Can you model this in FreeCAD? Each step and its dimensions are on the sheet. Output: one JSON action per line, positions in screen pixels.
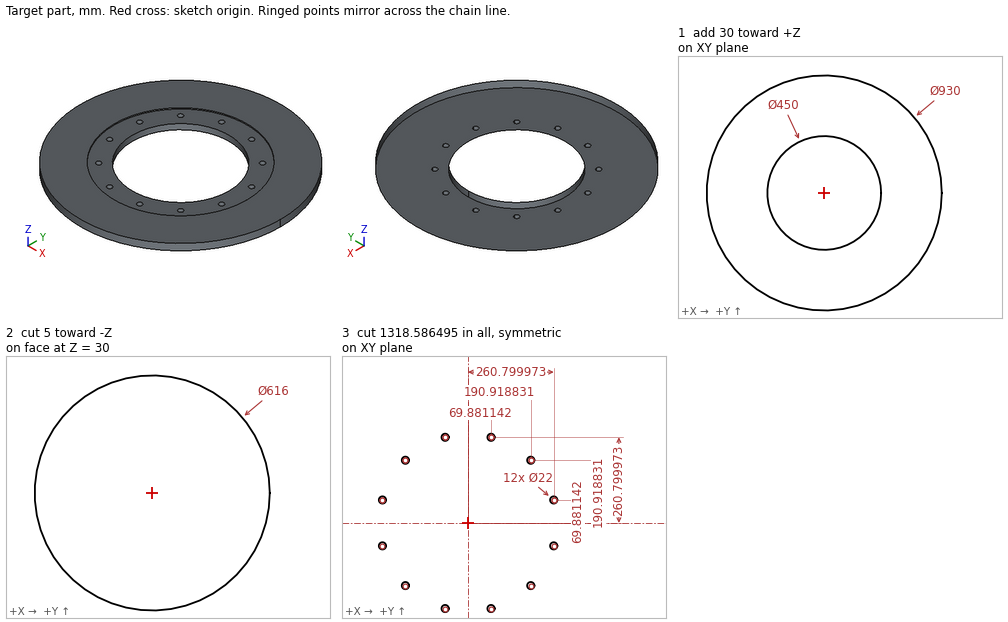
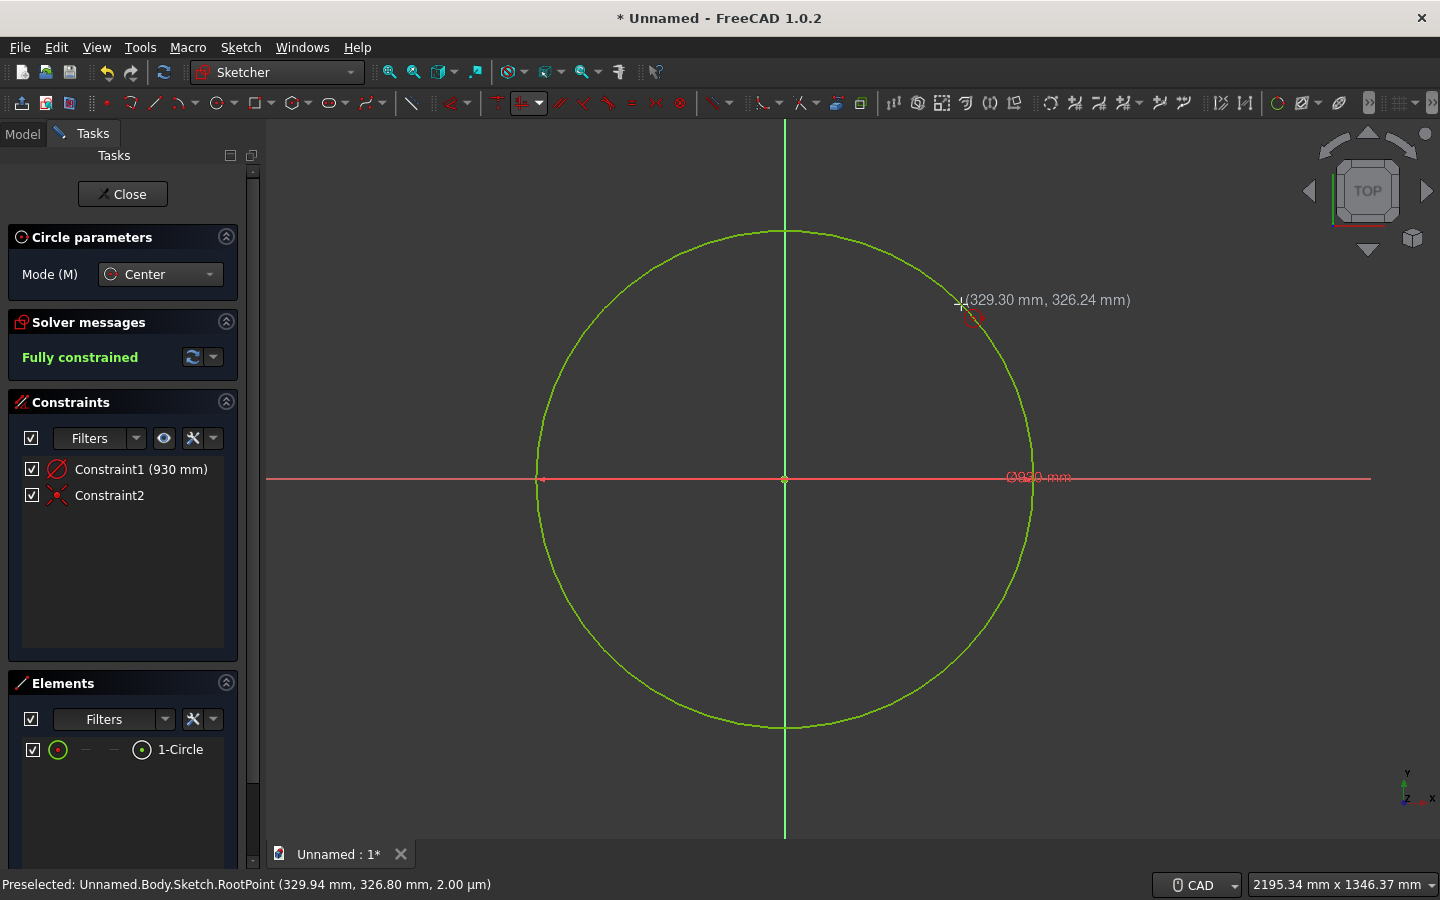
{"action": "left_click", "coordinate": [785, 479]}
{"action": "mouse_move", "coordinate": [870, 394]}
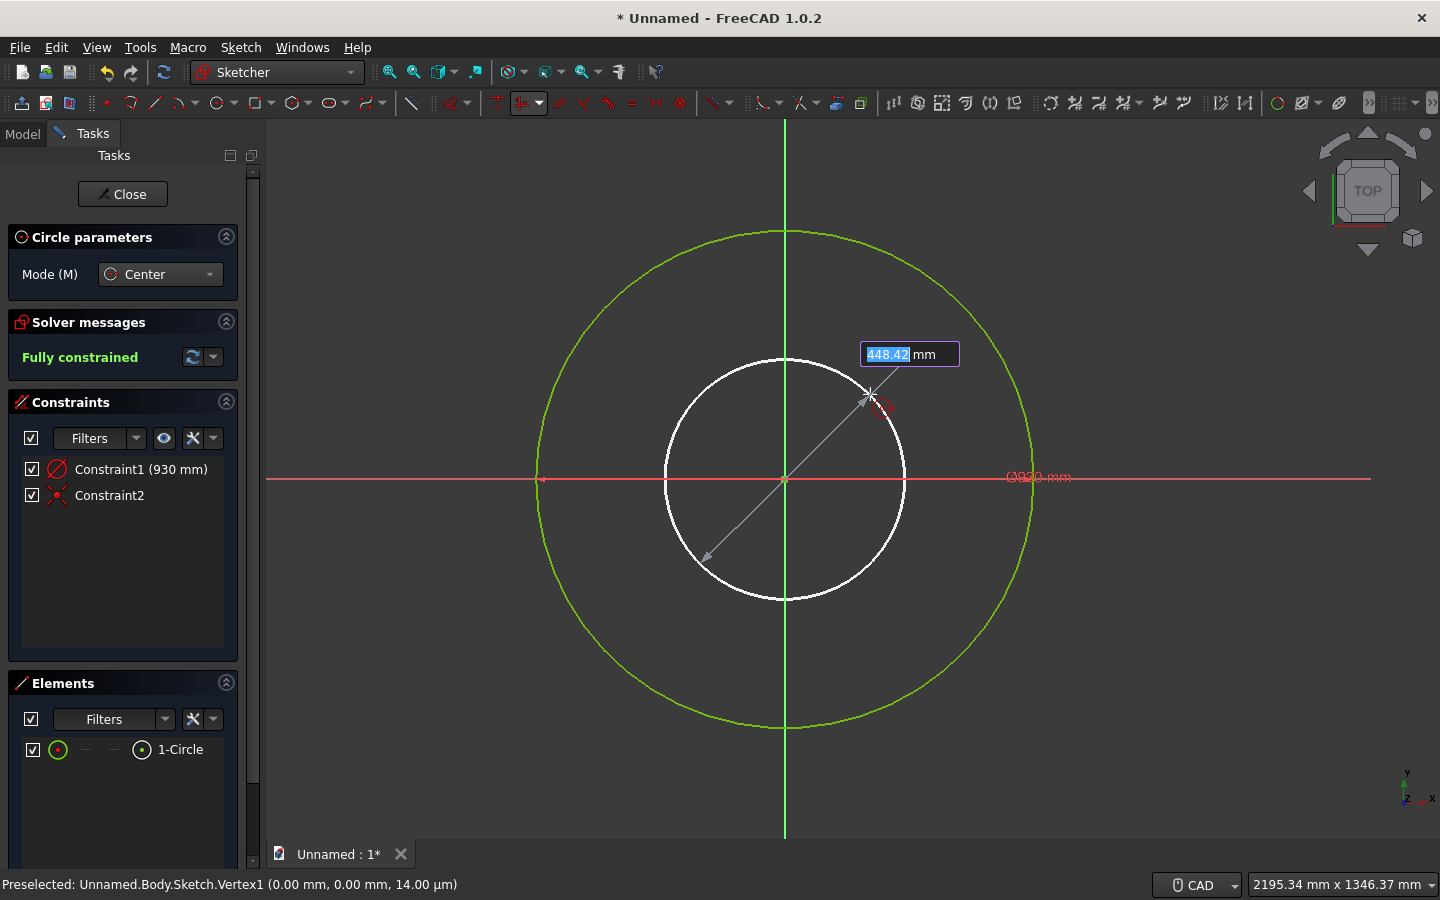
{"action": "type", "text": "450"}
{"action": "key", "text": "Return"}
{"action": "key", "text": "Escape"}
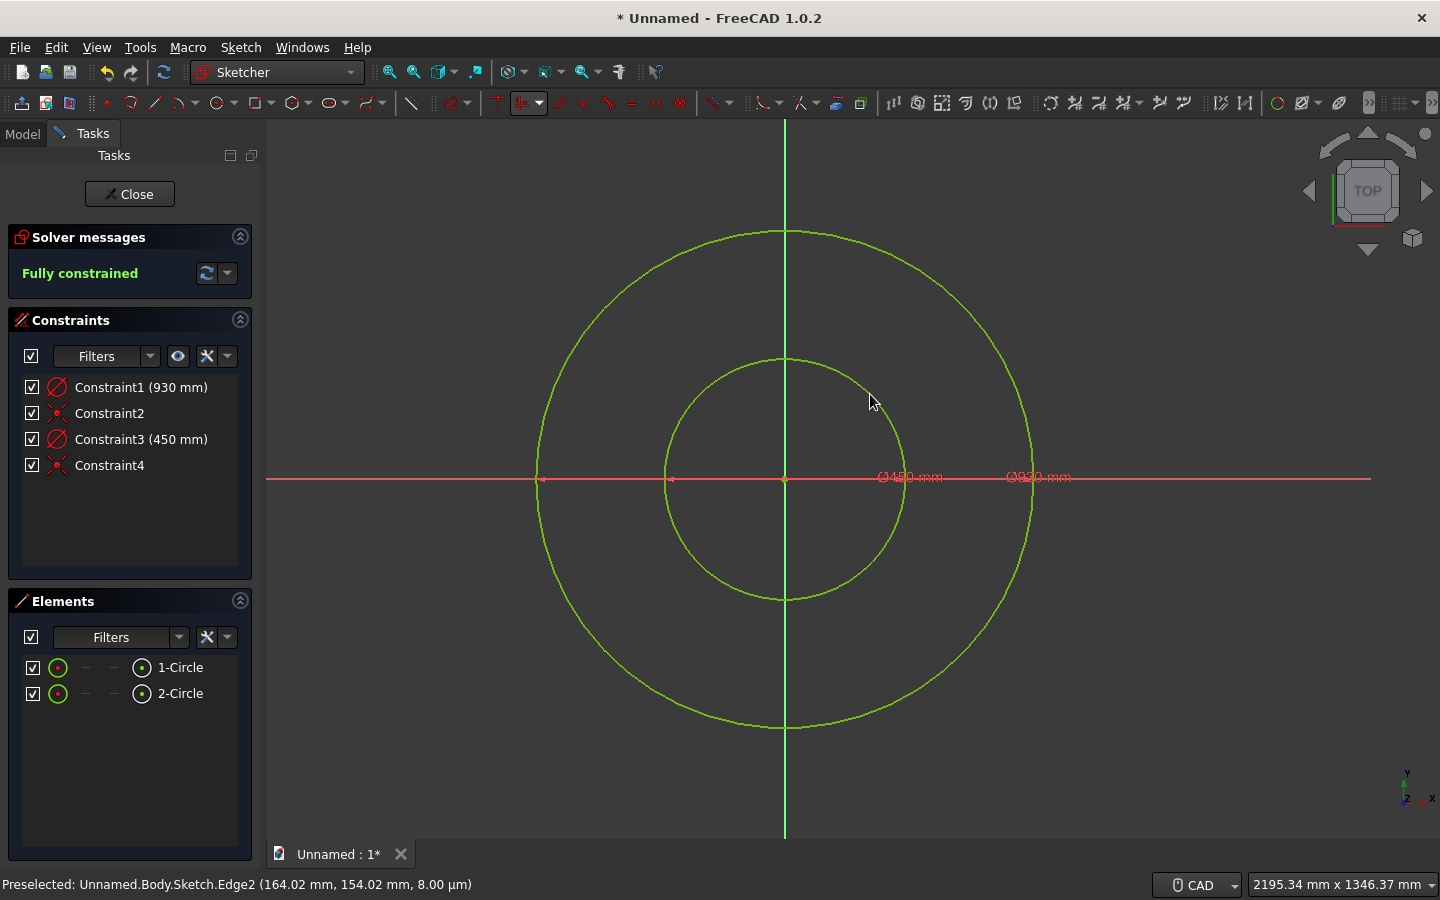
{"action": "left_click", "coordinate": [130, 194]}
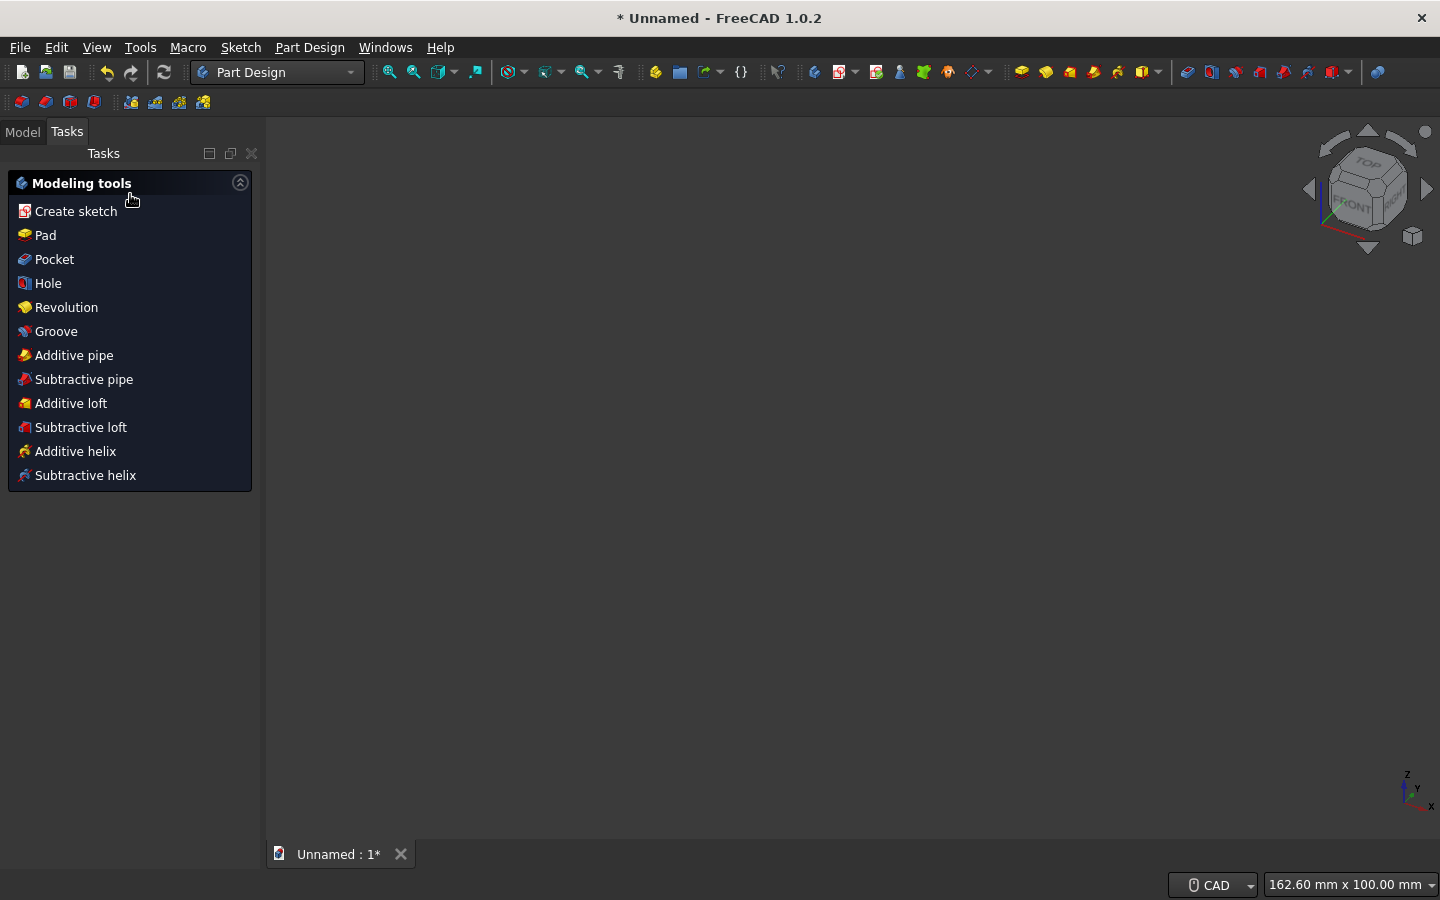
{"action": "left_click", "coordinate": [1022, 72]}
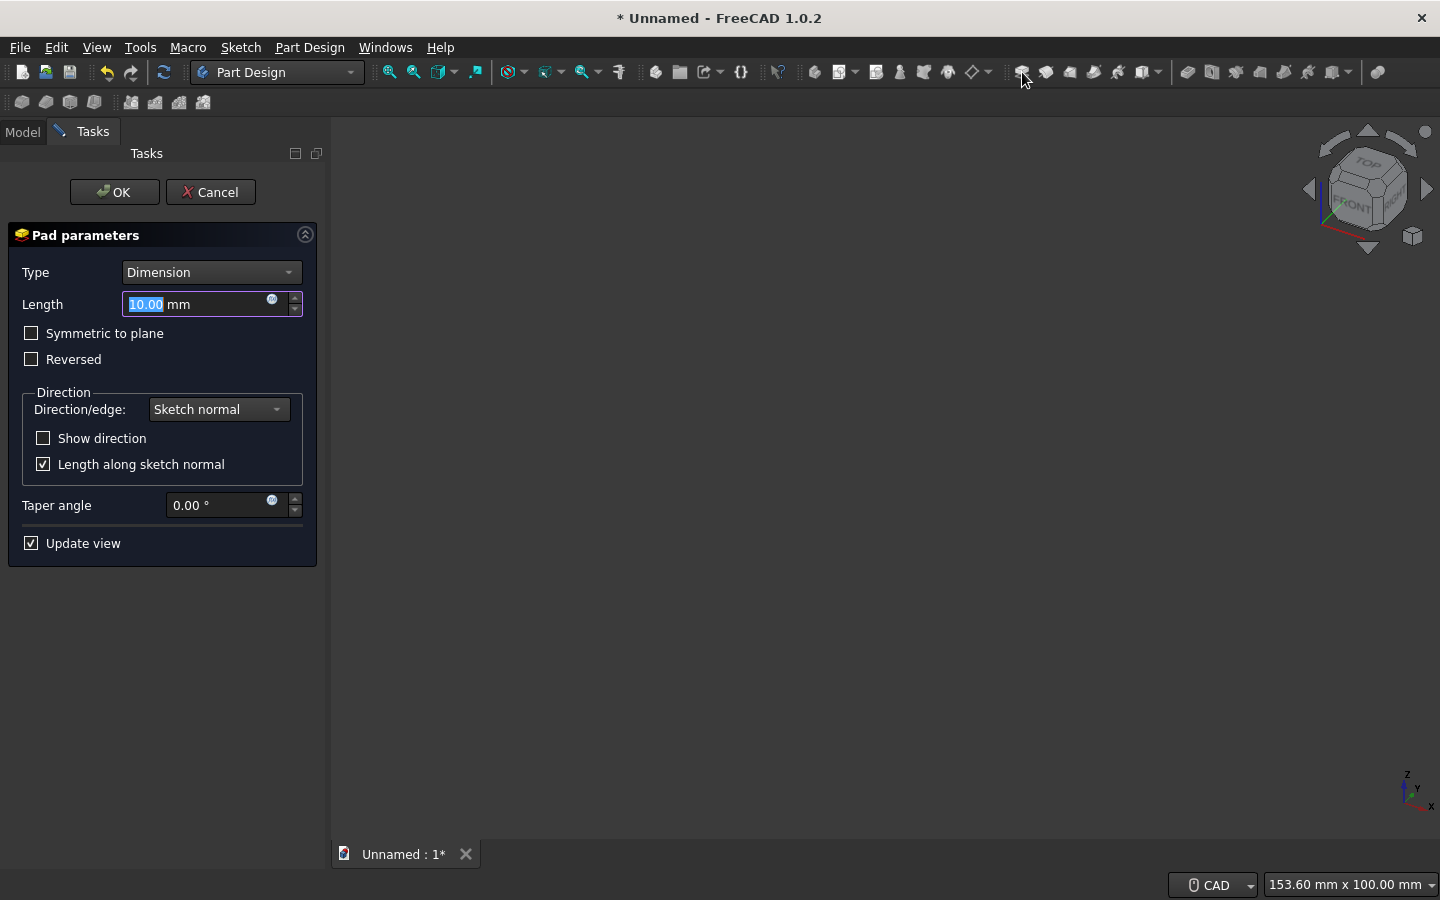
{"action": "type", "text": "30"}
{"action": "key", "text": "Tab"}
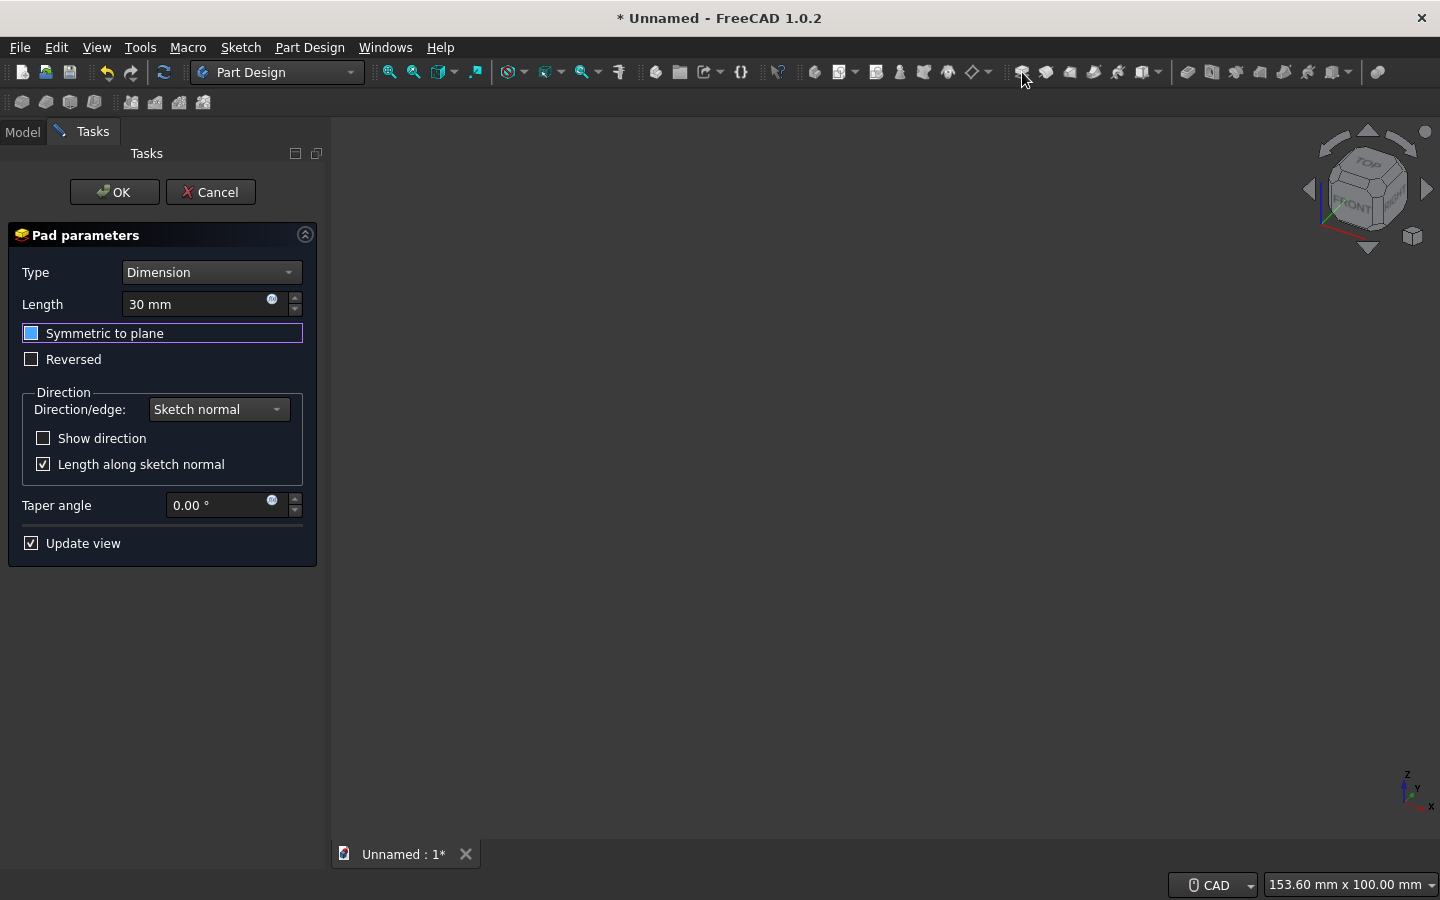
{"action": "left_click", "coordinate": [115, 192]}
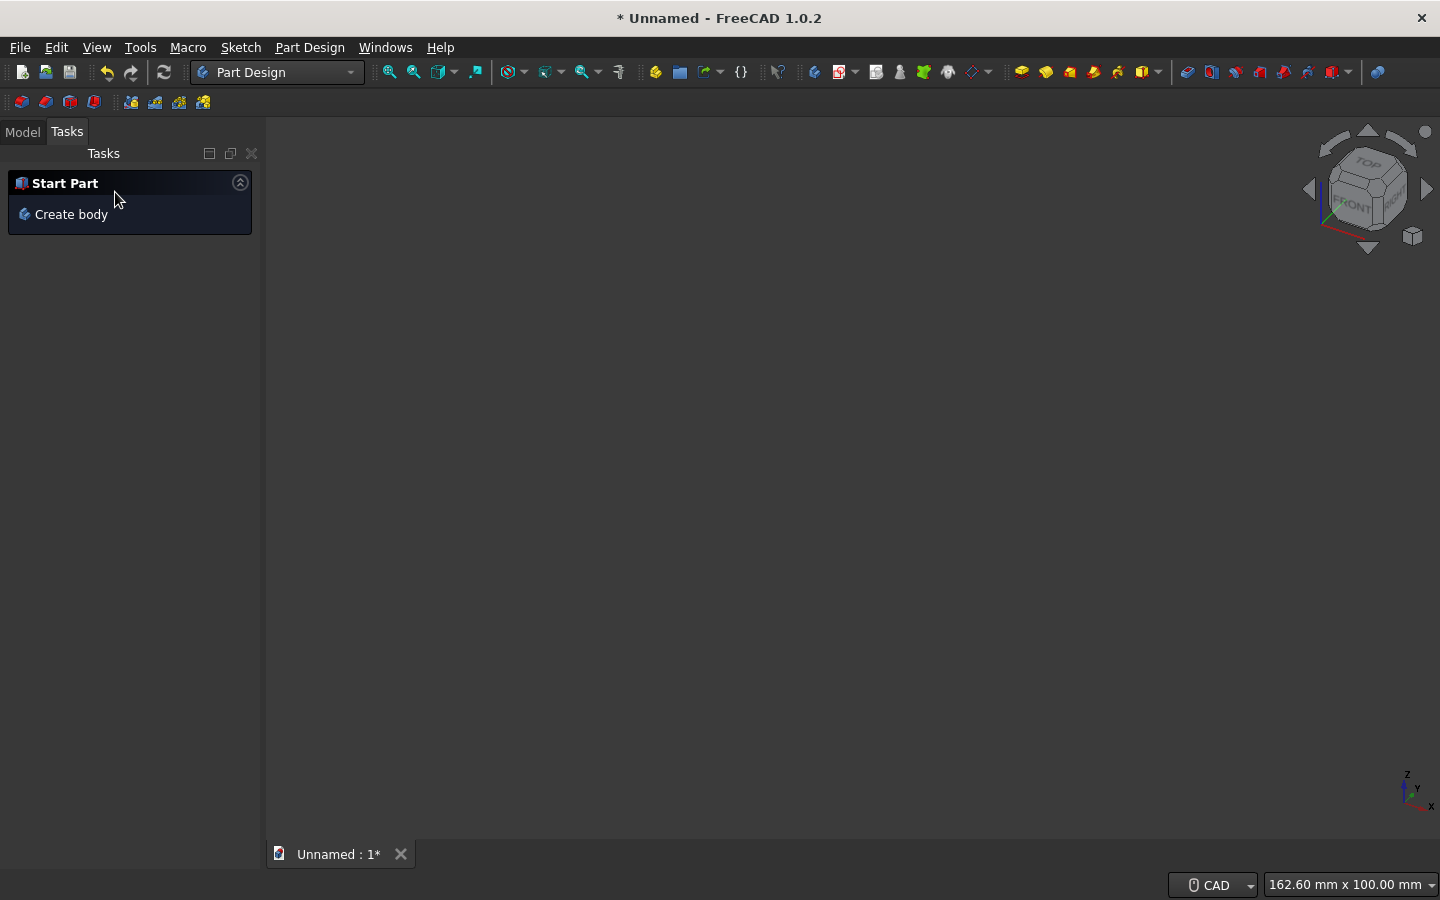
{"action": "left_click", "coordinate": [390, 72]}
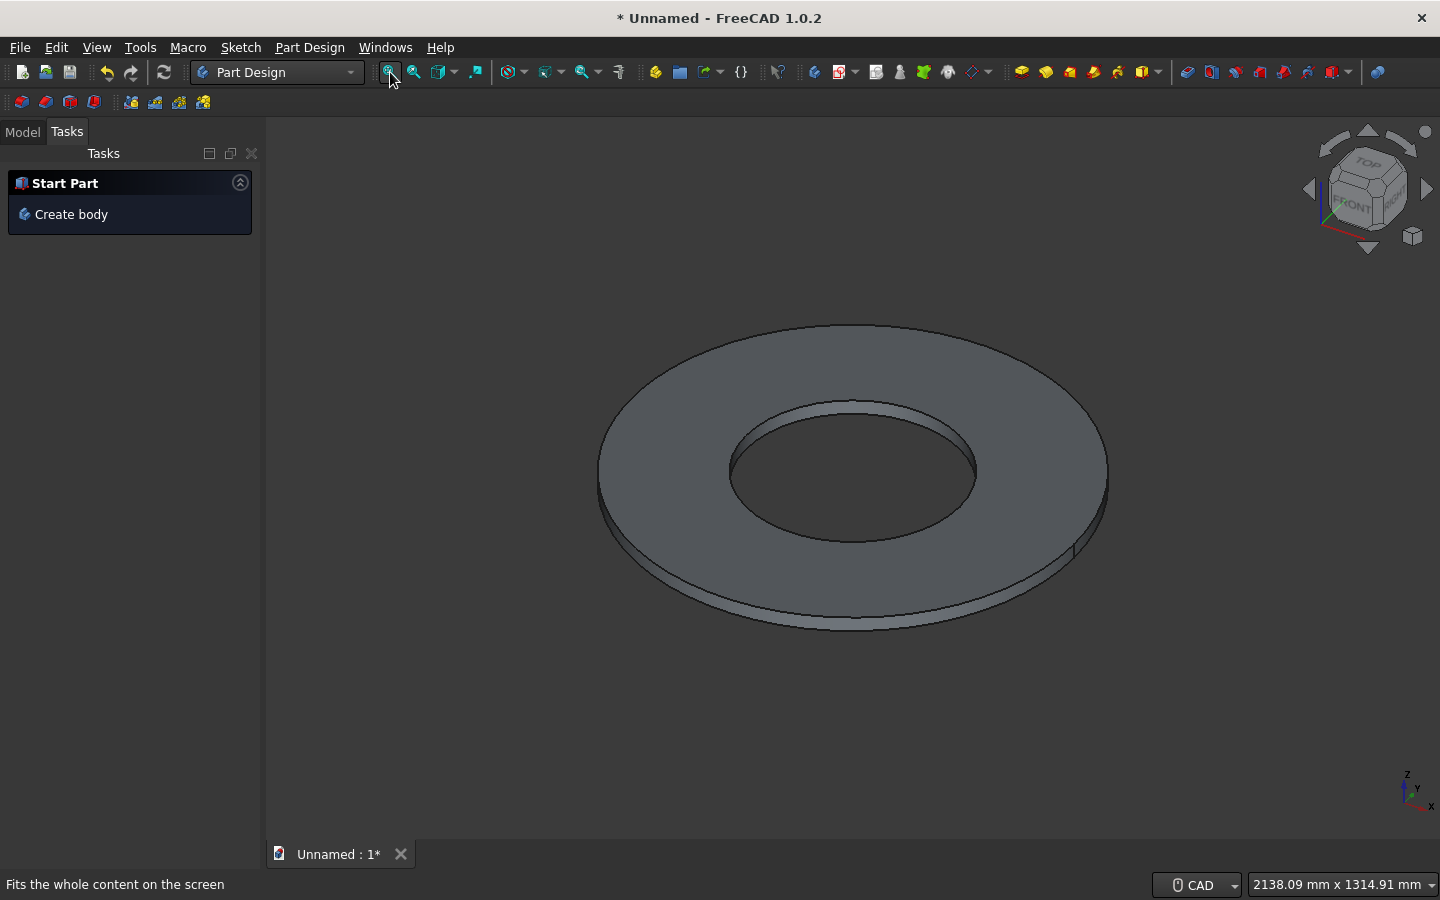
{"action": "left_click", "coordinate": [1052, 440]}